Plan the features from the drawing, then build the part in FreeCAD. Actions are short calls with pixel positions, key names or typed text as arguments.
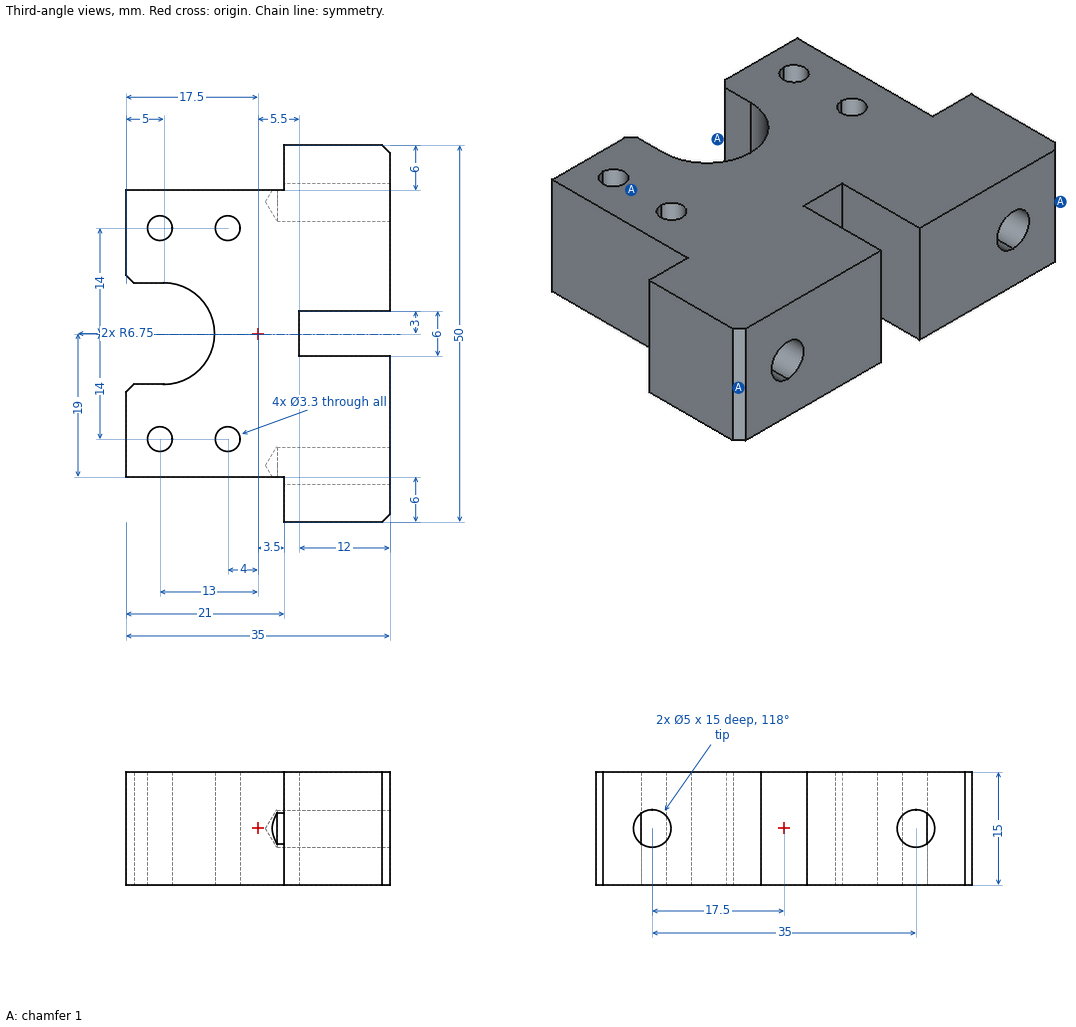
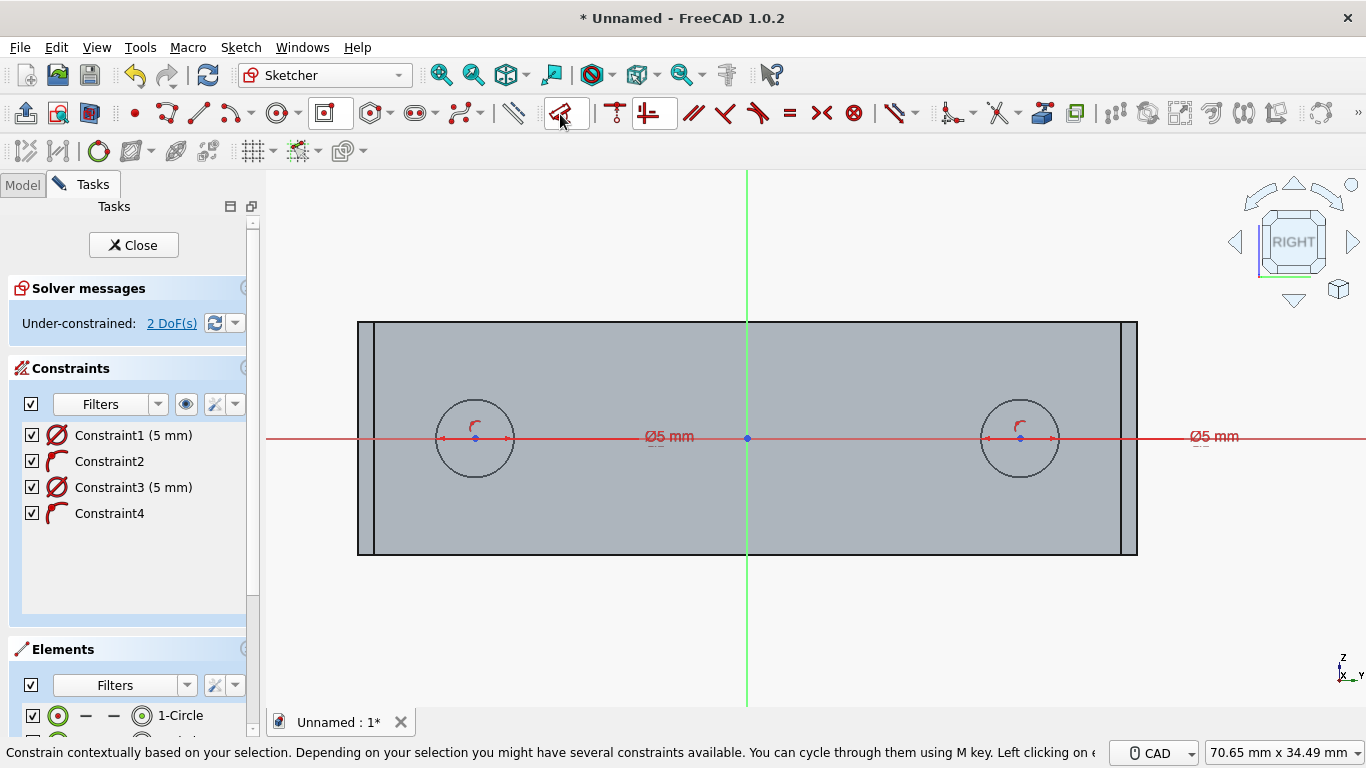
click(475, 438)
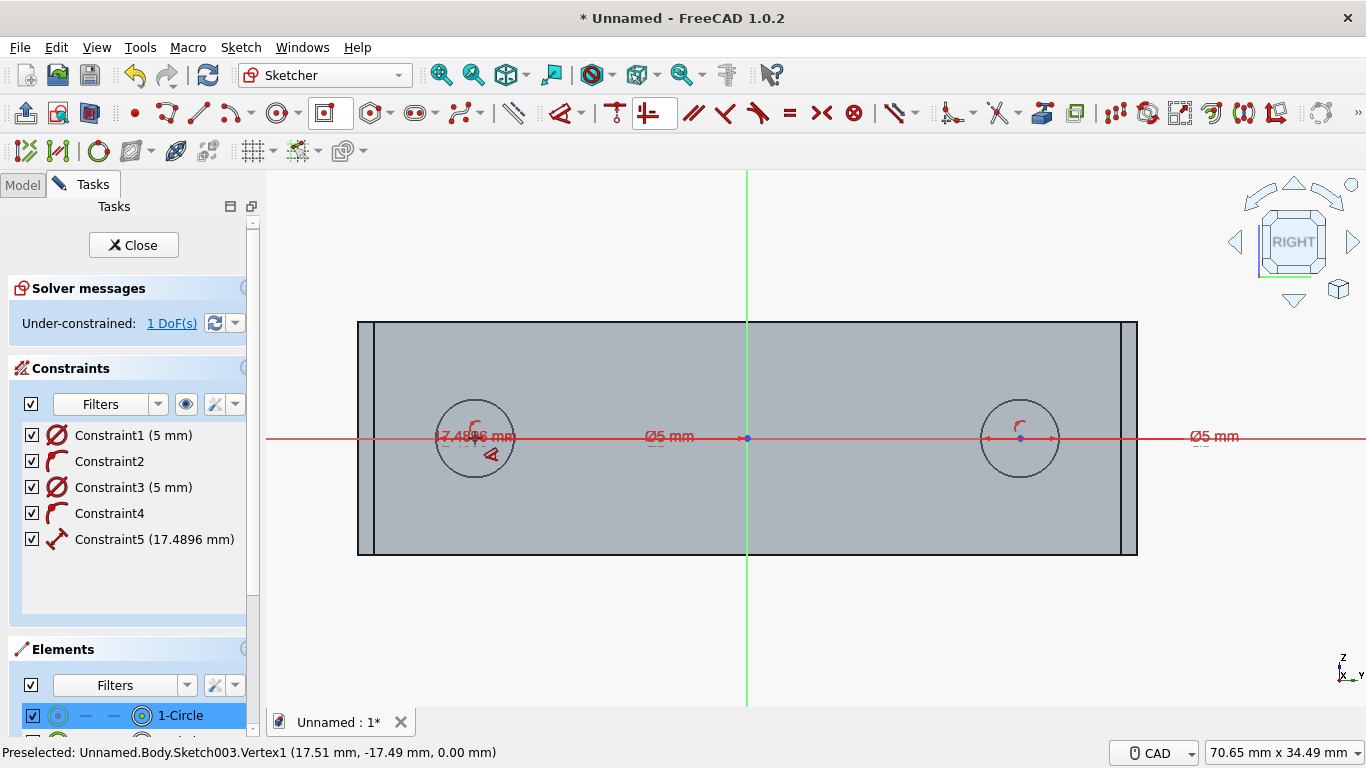
click(1020, 438)
click(622, 472)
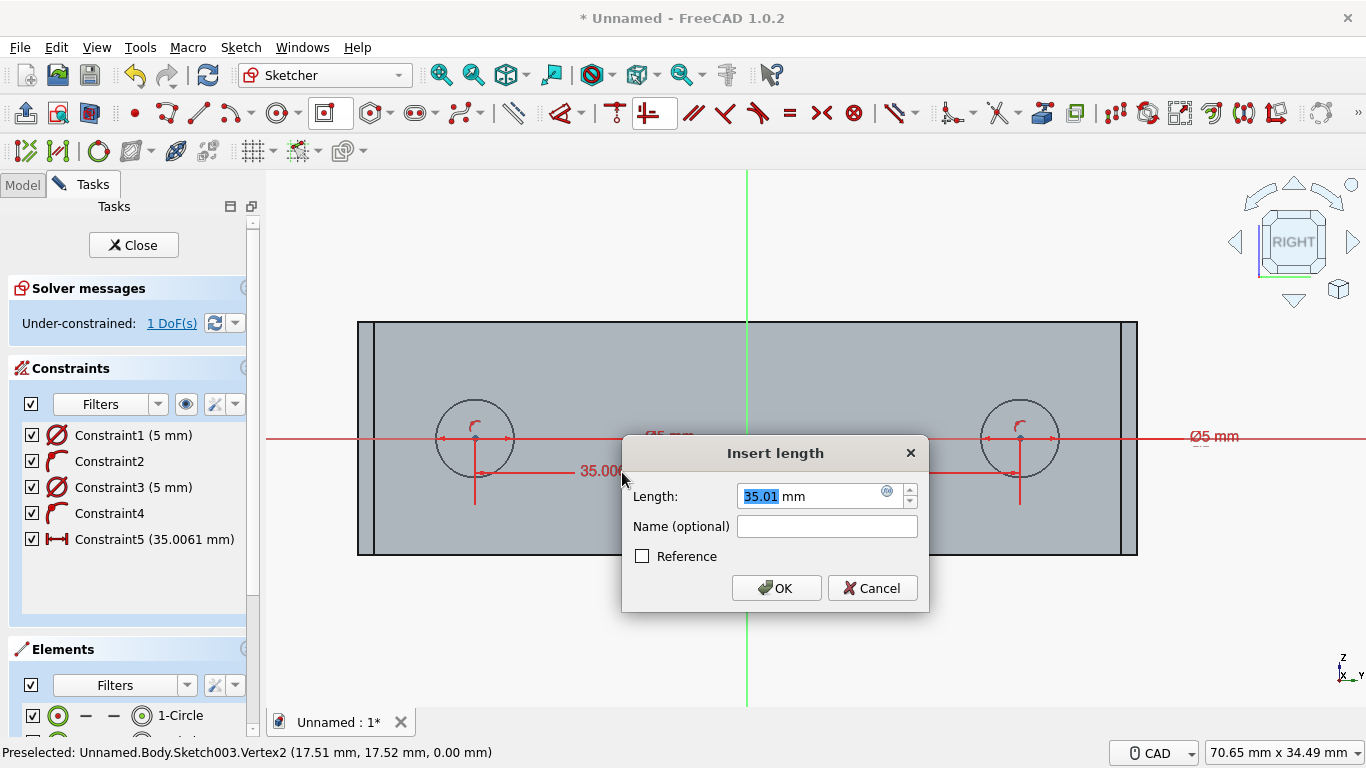
text(35)
key(Return)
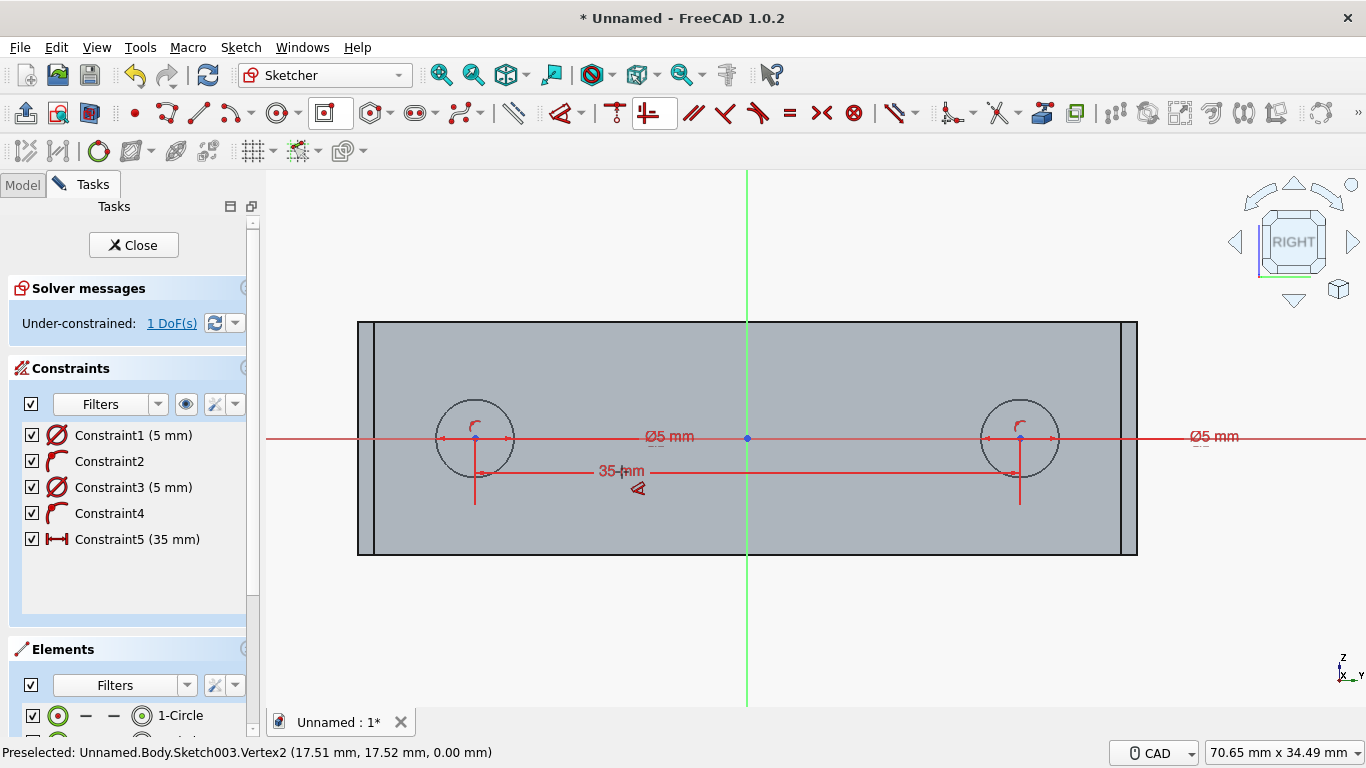
click(475, 438)
click(549, 472)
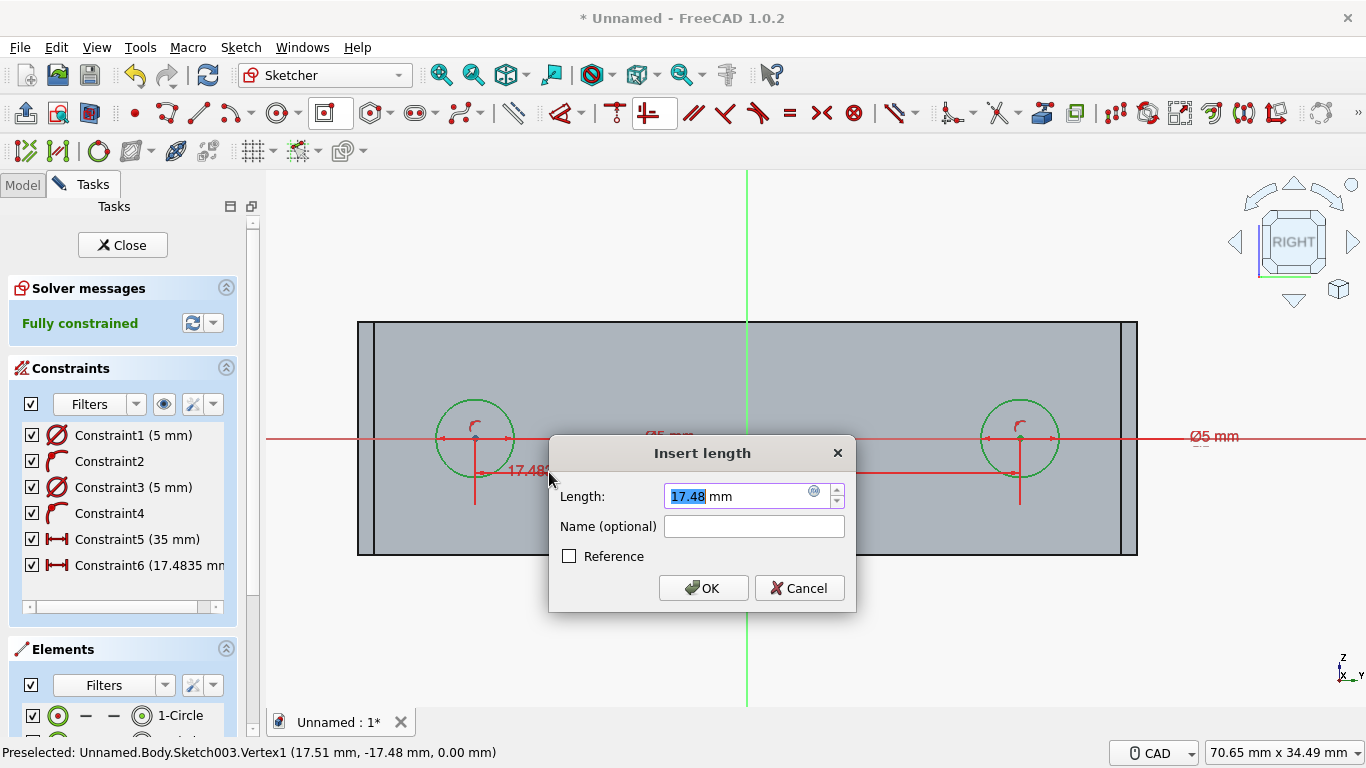
text(17.5)
key(Return)
key(Escape)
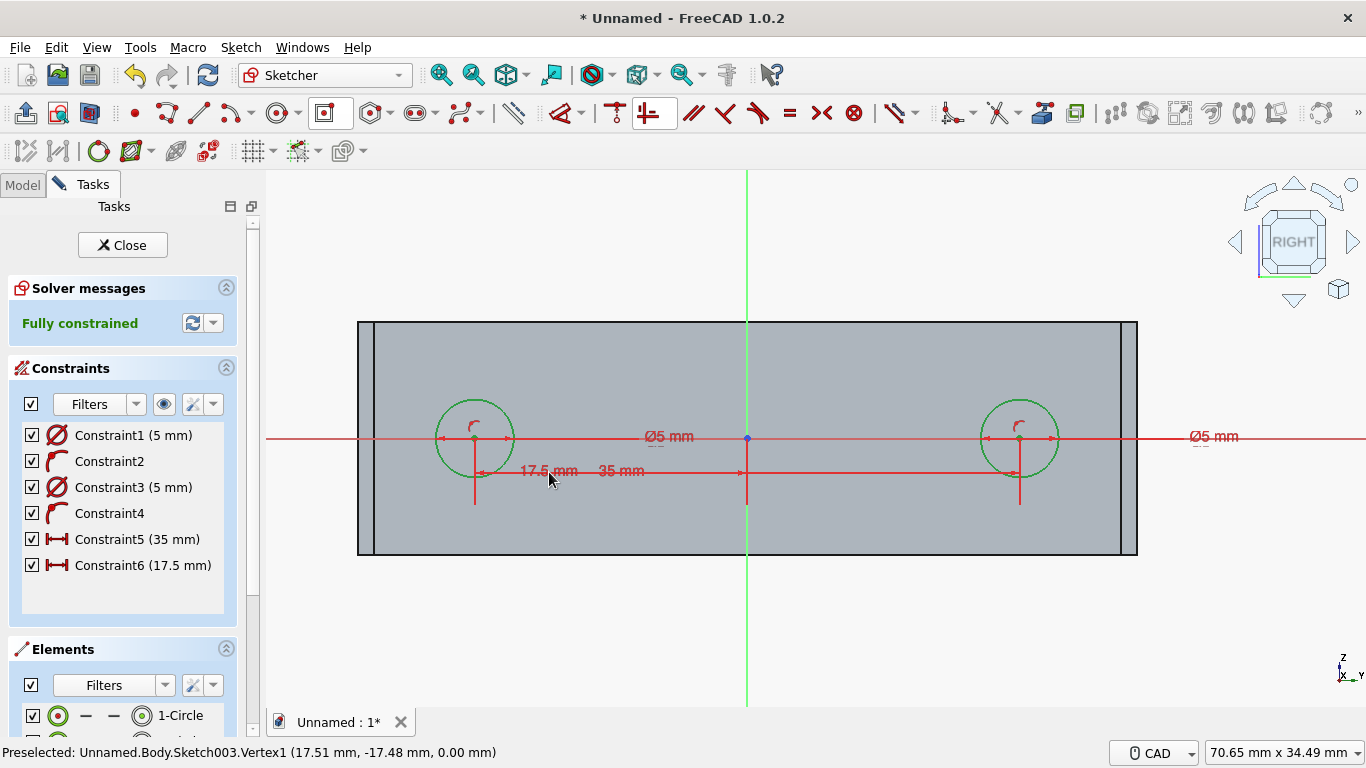
click(123, 245)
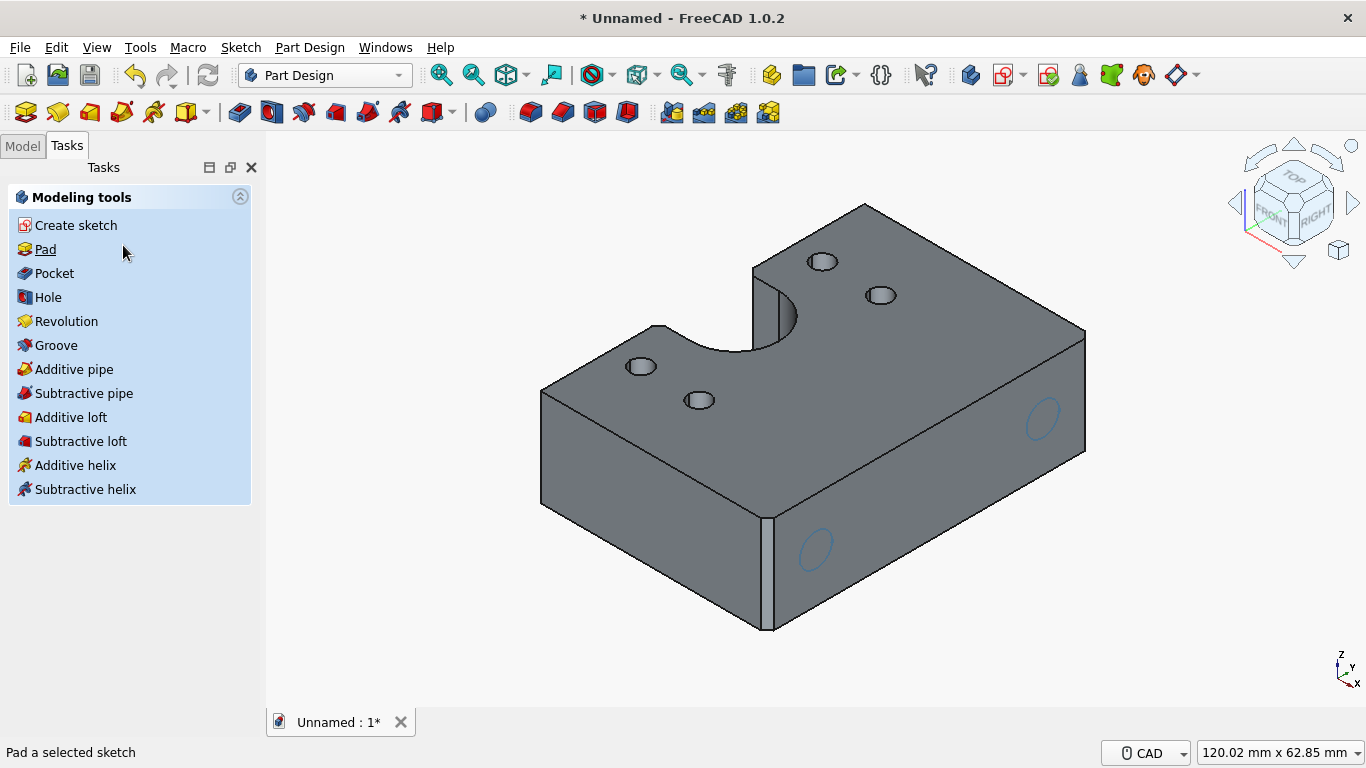
click(272, 112)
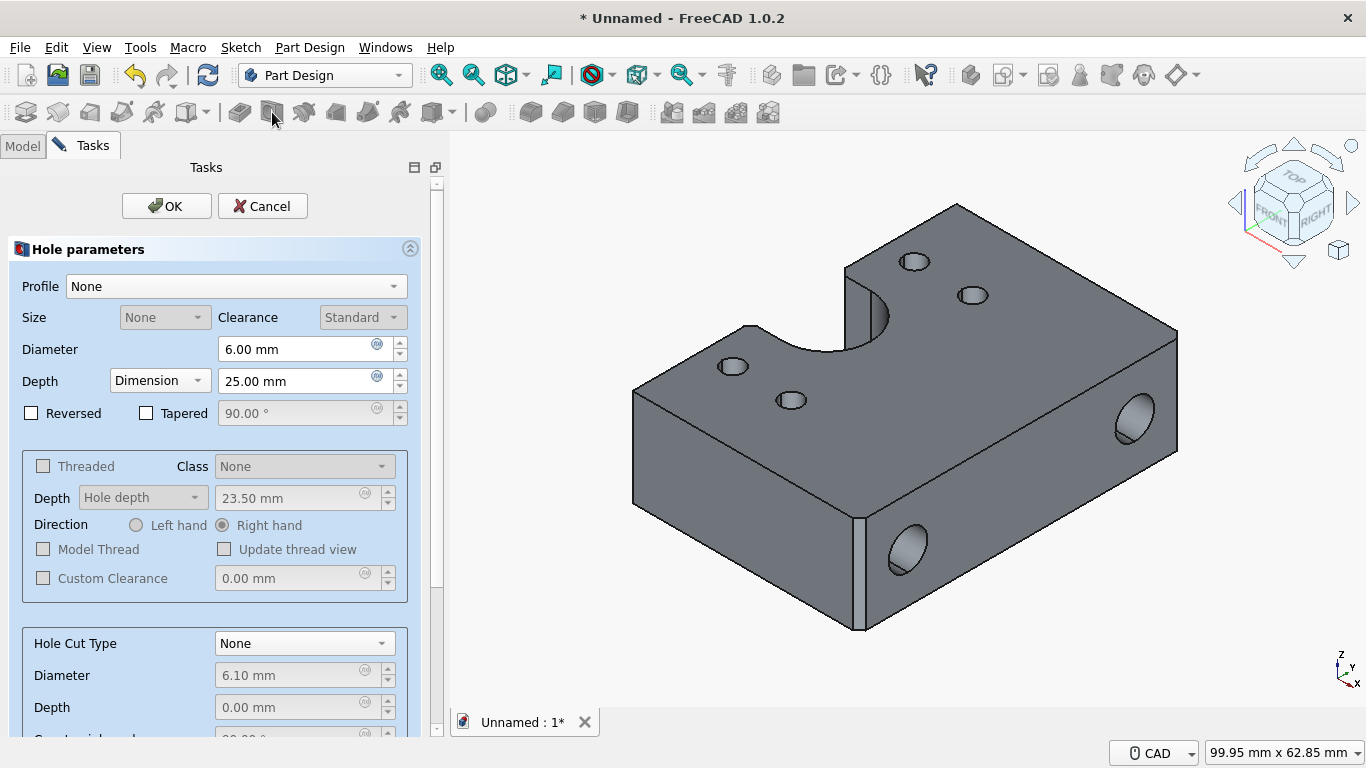
triple_click(305, 349)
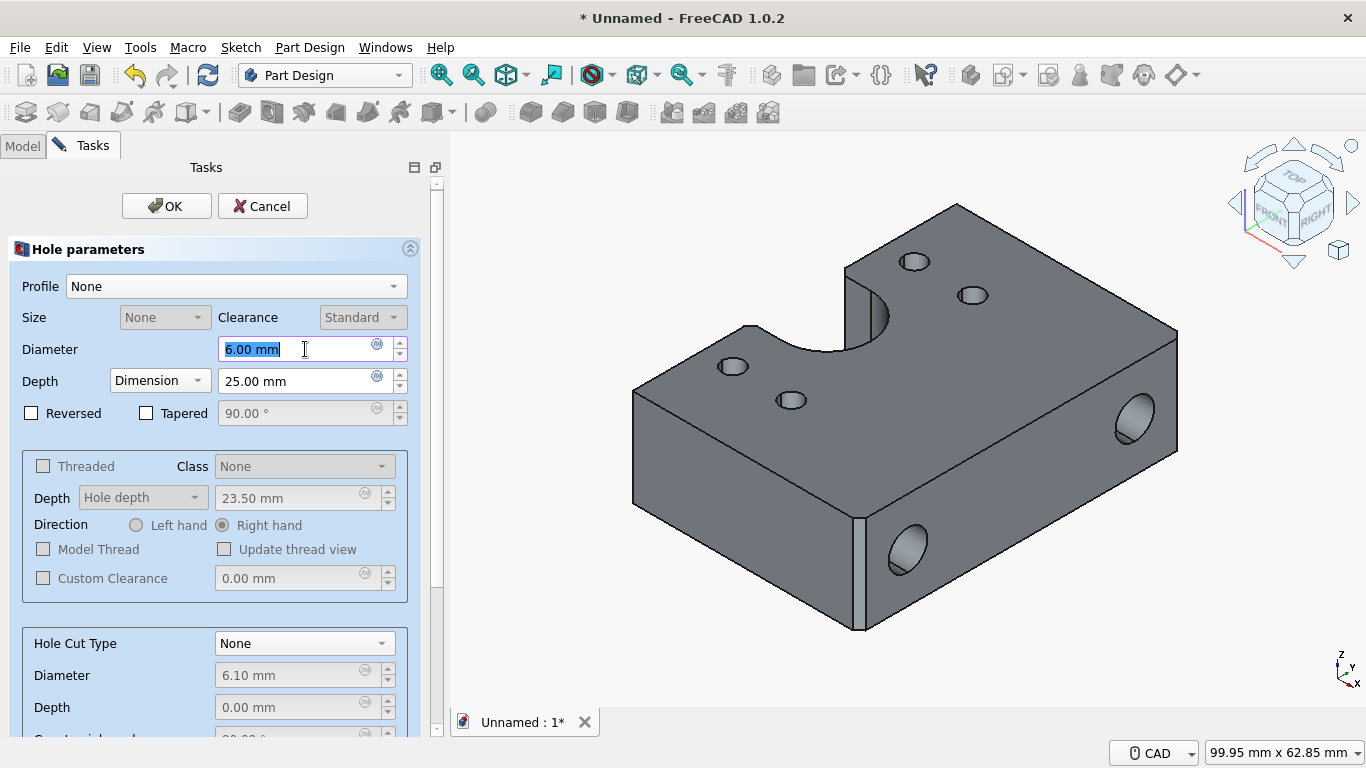
text(5)
key(Tab)